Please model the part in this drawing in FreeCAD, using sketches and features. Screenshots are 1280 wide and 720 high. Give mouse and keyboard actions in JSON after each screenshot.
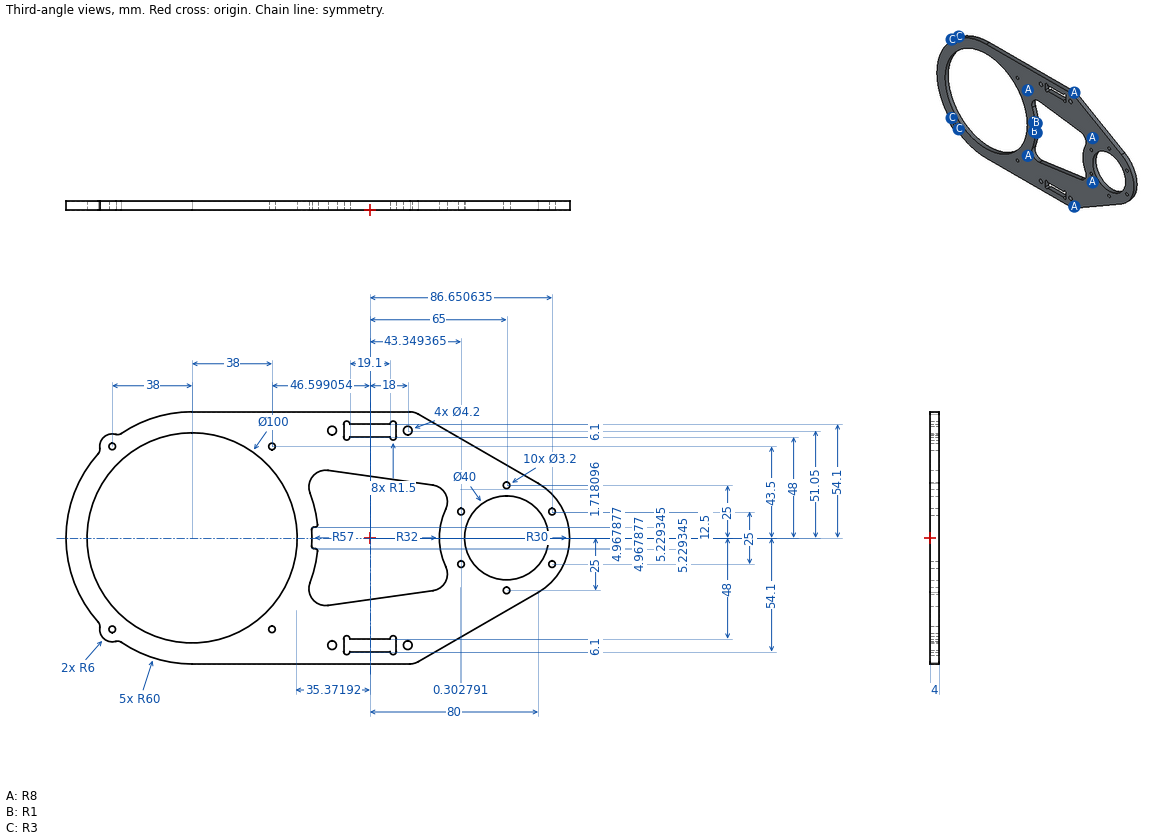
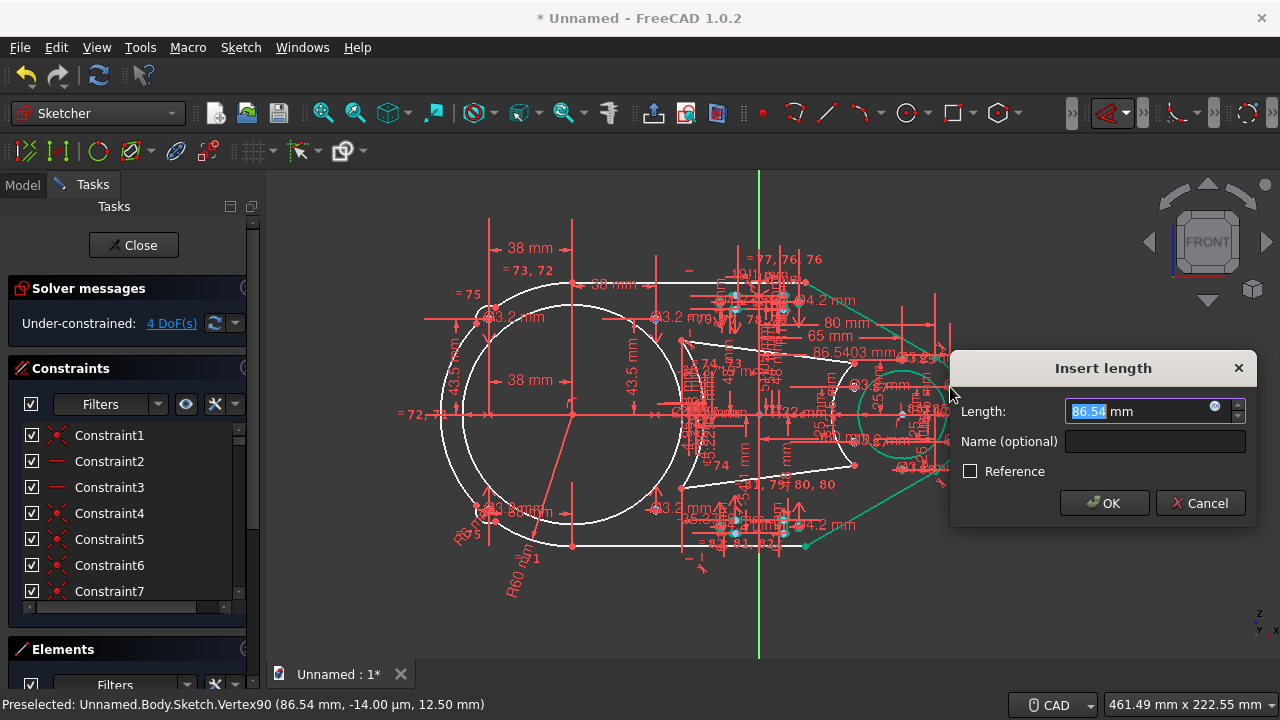
{"action": "type", "text": "86.650635"}
{"action": "key", "text": "Return"}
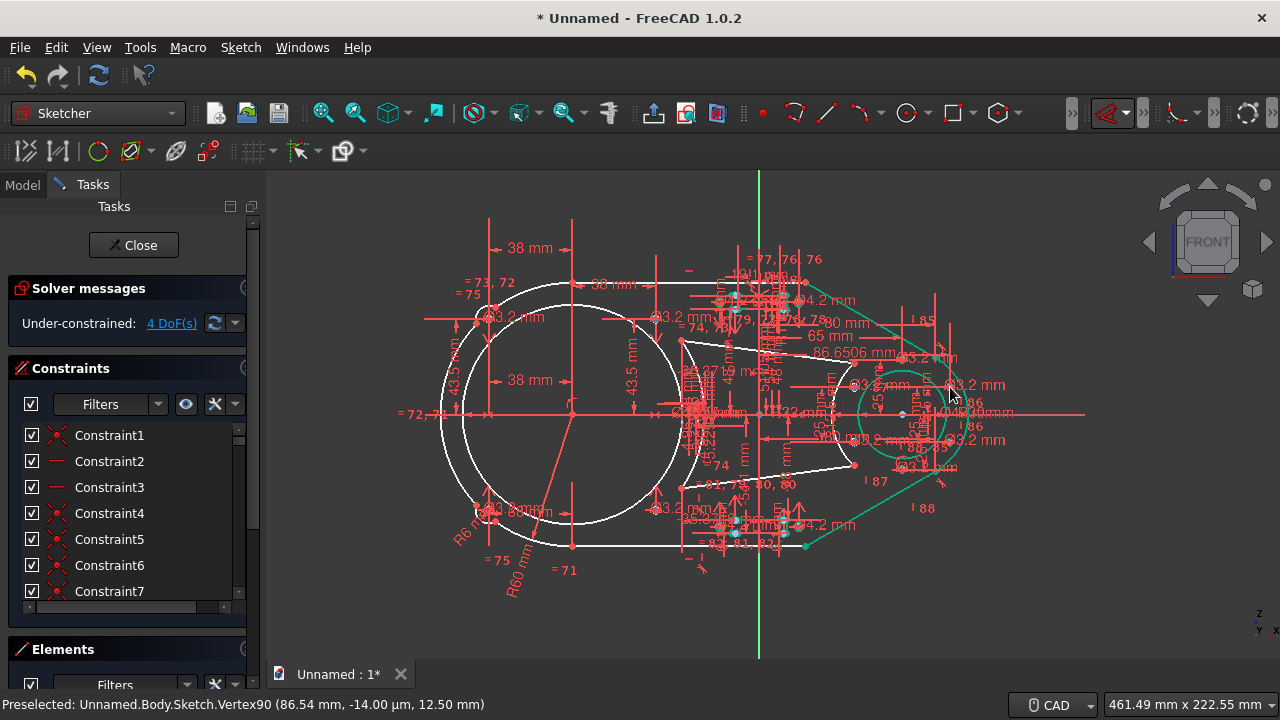
{"action": "left_click", "coordinate": [855, 387]}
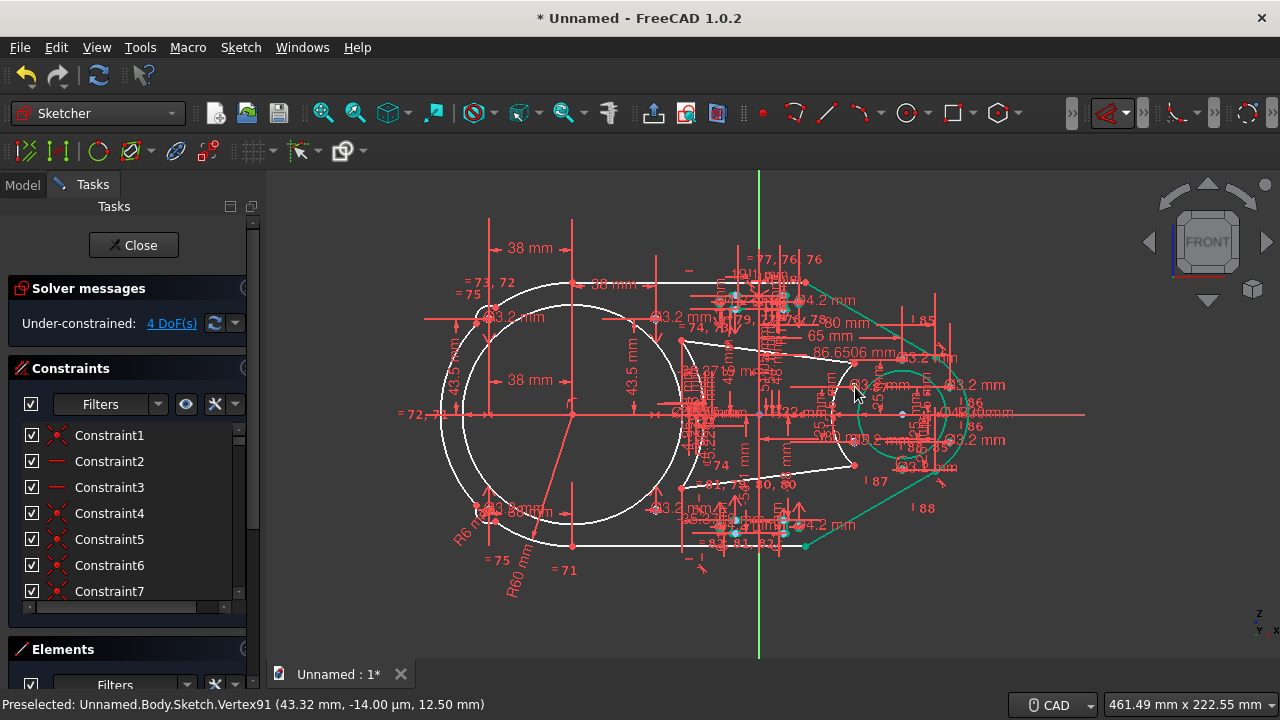
{"action": "key", "text": "l"}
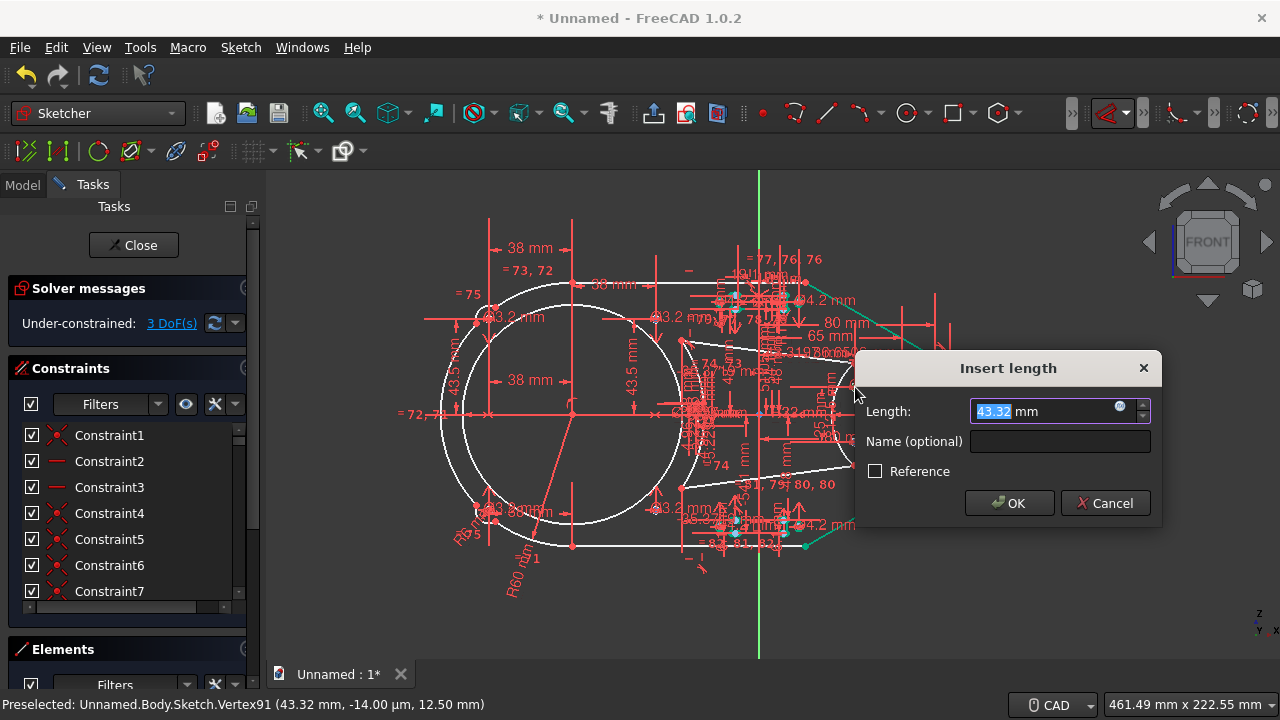
{"action": "type", "text": "43.349365"}
{"action": "key", "text": "Return"}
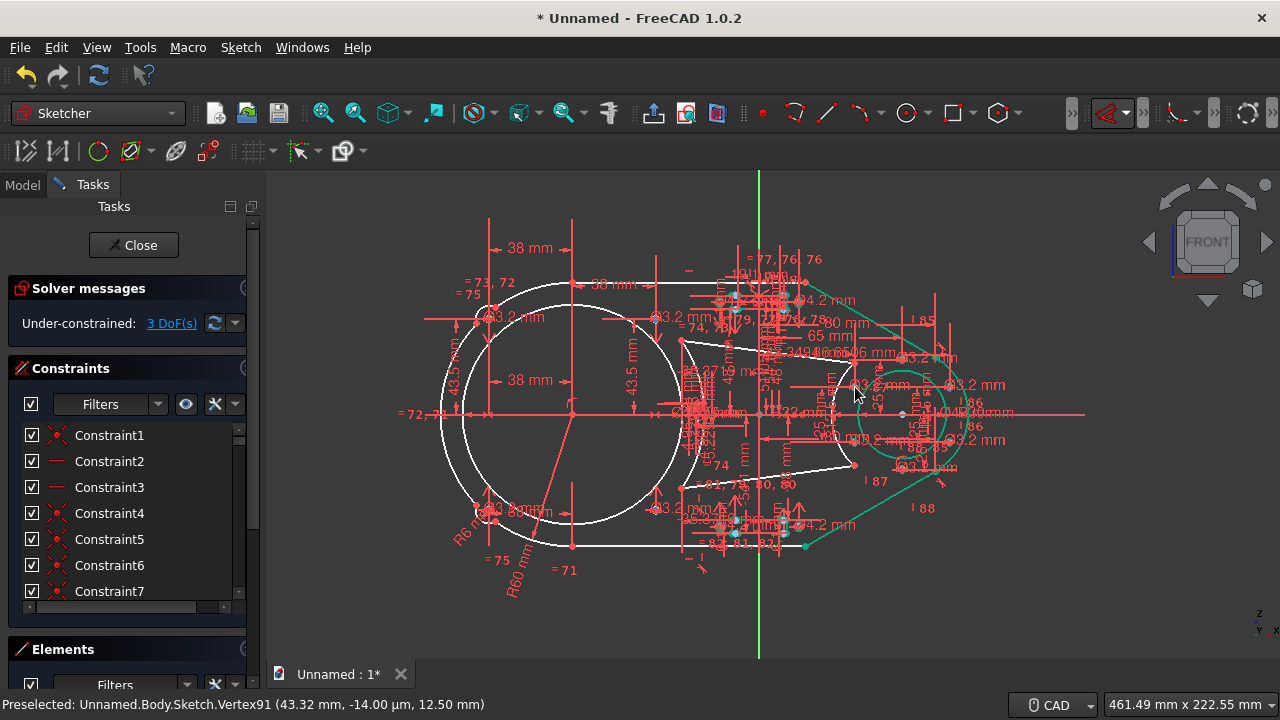
{"action": "left_click", "coordinate": [656, 319]}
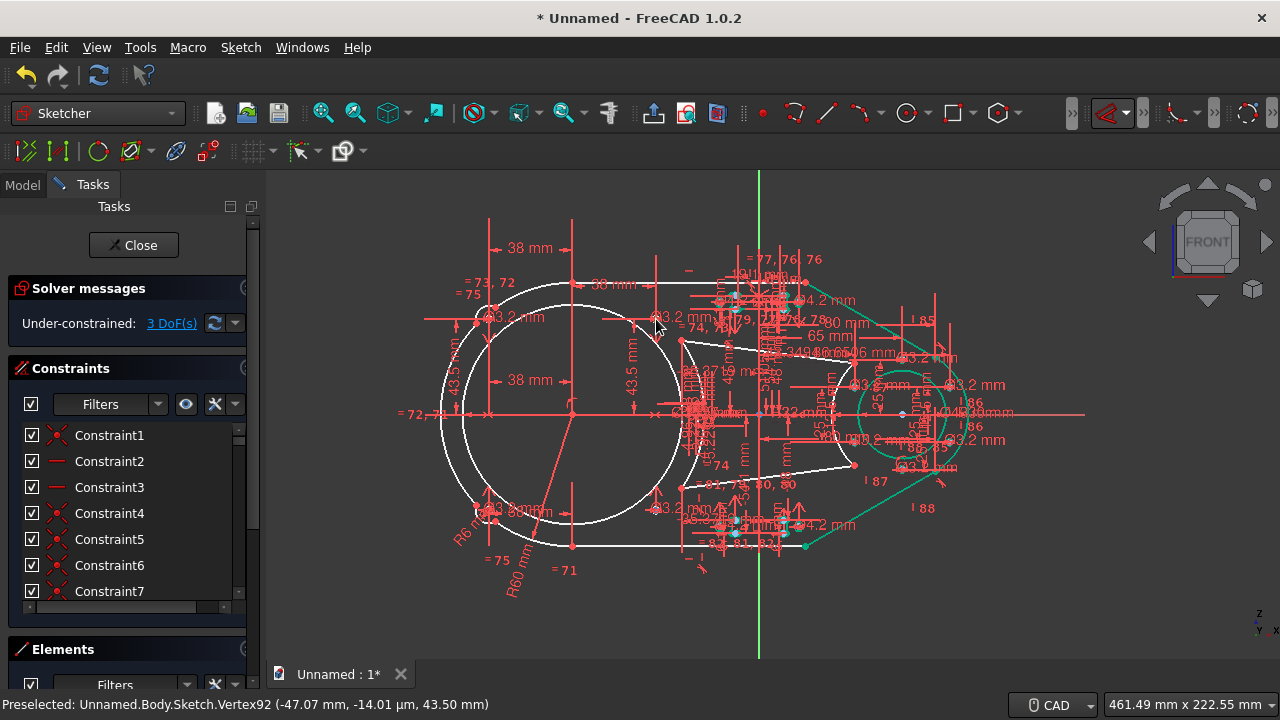
{"action": "key", "text": "l"}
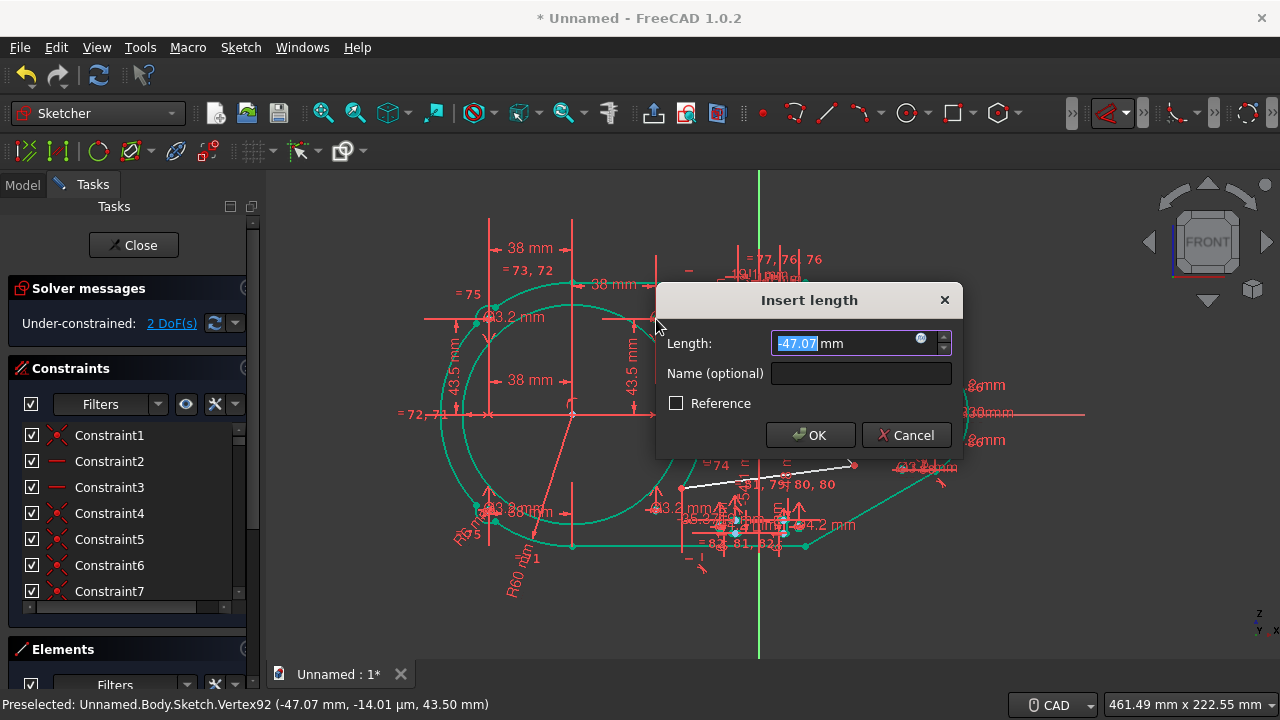
{"action": "type", "text": "-46.599054"}
{"action": "key", "text": "Return"}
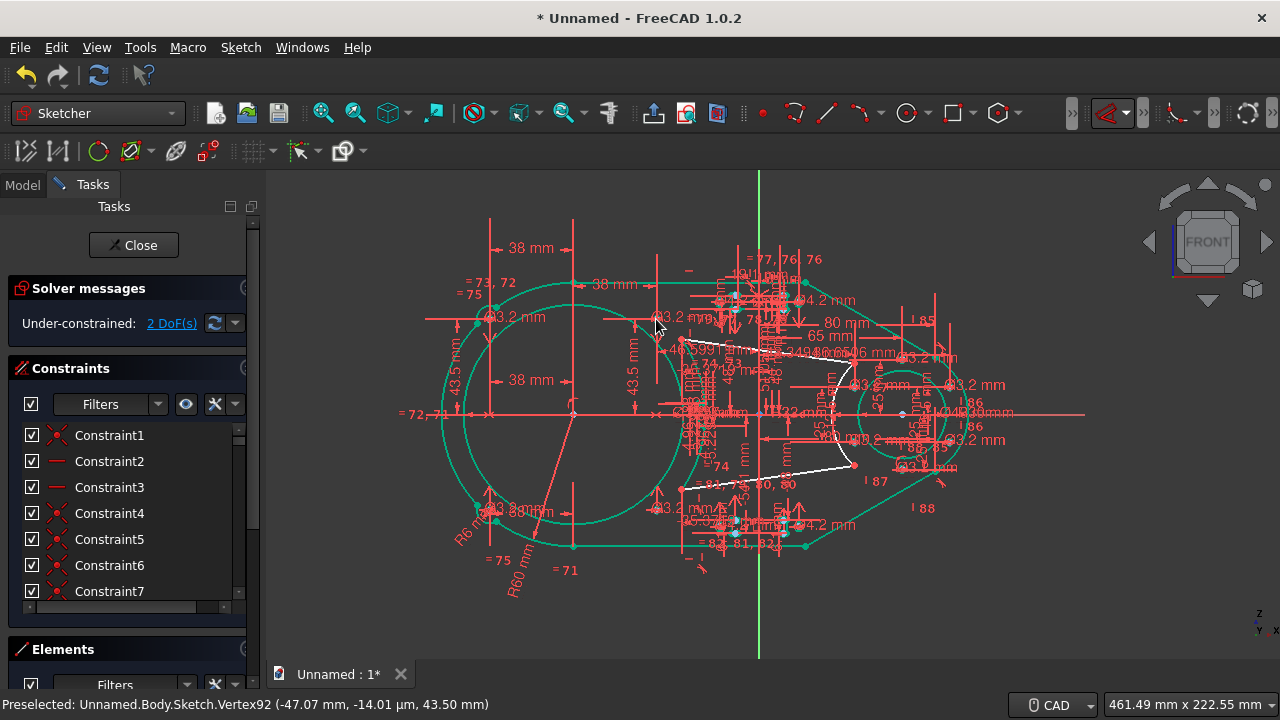
{"action": "scroll", "coordinate": [854, 363], "scroll_direction": "up", "scroll_amount": 12}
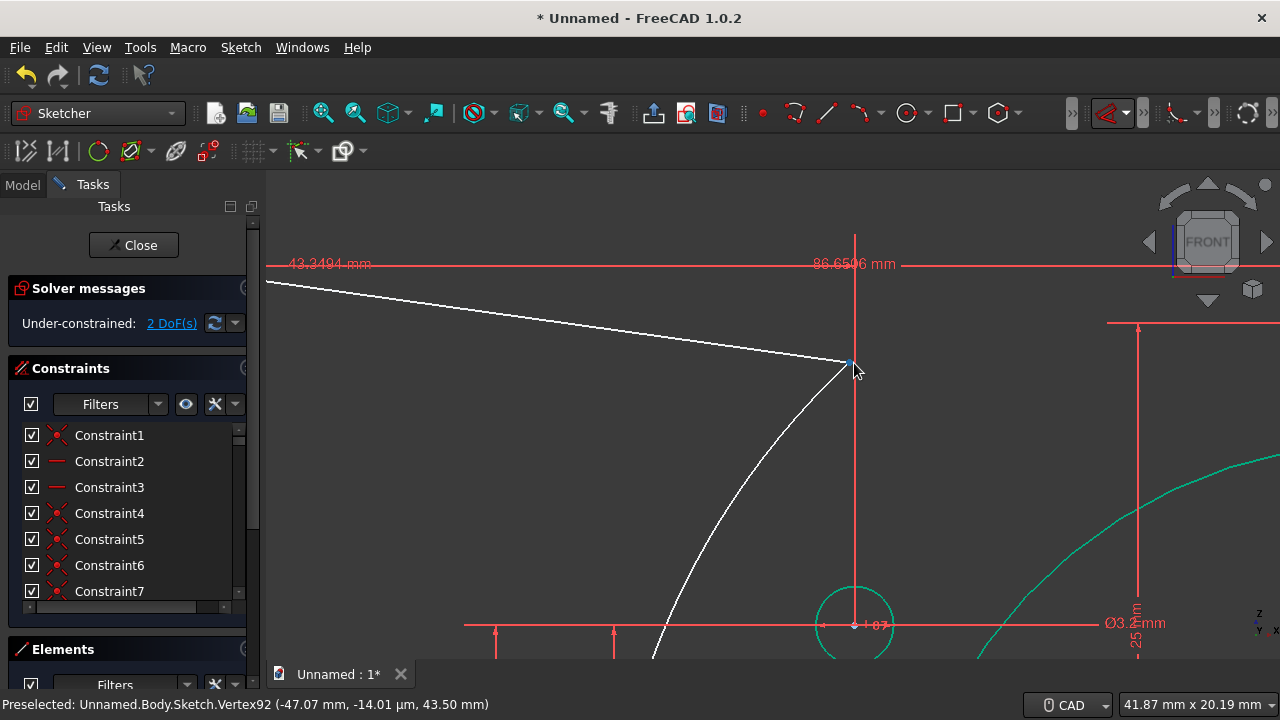
{"action": "left_click", "coordinate": [849, 363]}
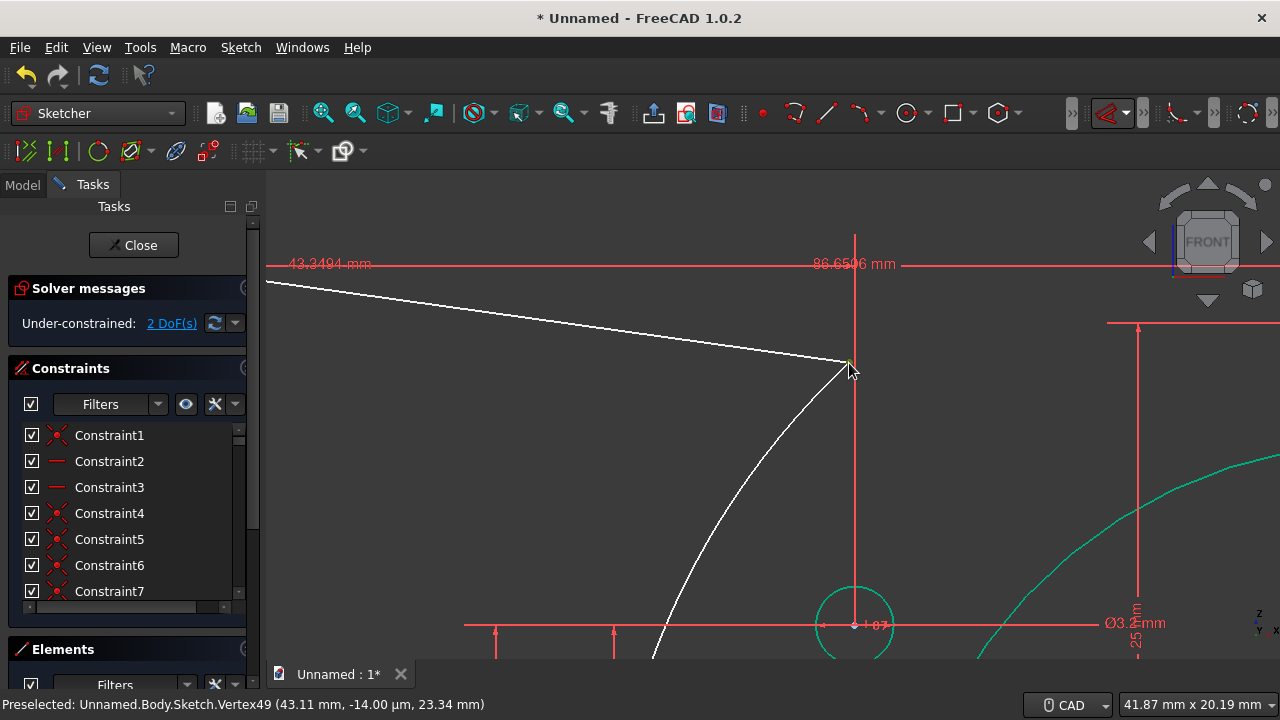
{"action": "scroll", "coordinate": [854, 363], "scroll_direction": "down", "scroll_amount": 12}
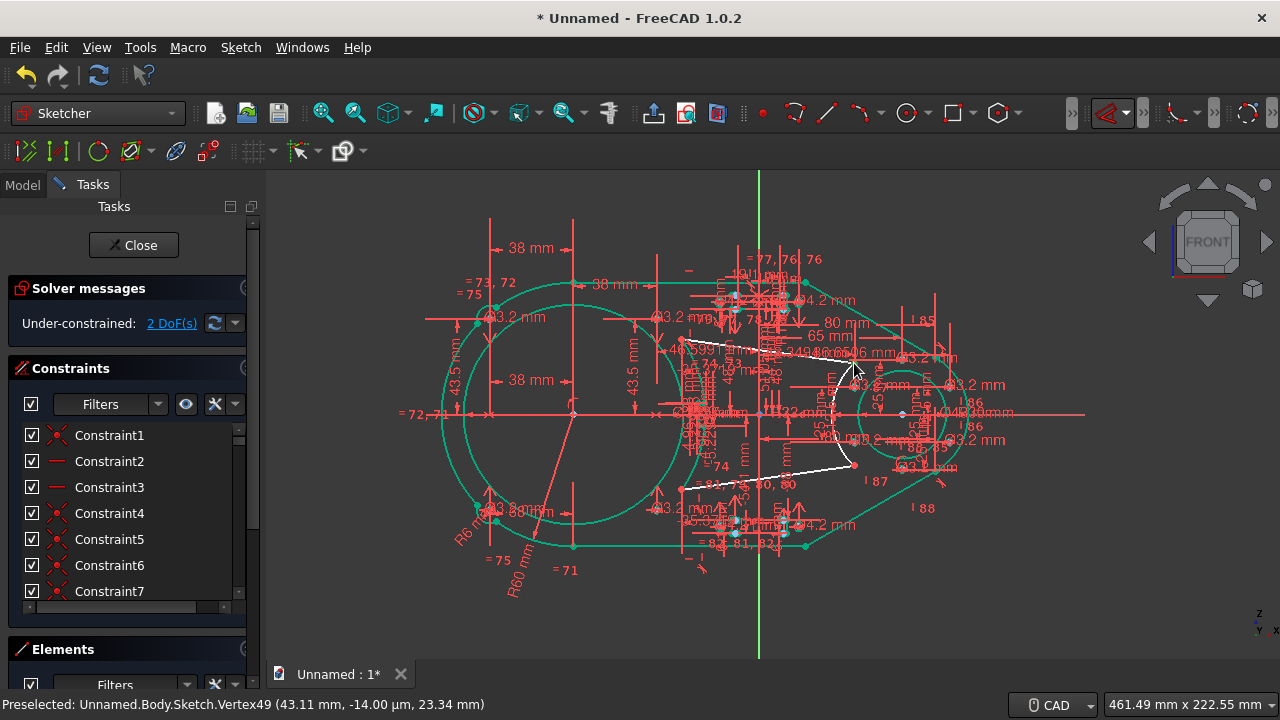
{"action": "scroll", "coordinate": [902, 360], "scroll_direction": "up", "scroll_amount": 12}